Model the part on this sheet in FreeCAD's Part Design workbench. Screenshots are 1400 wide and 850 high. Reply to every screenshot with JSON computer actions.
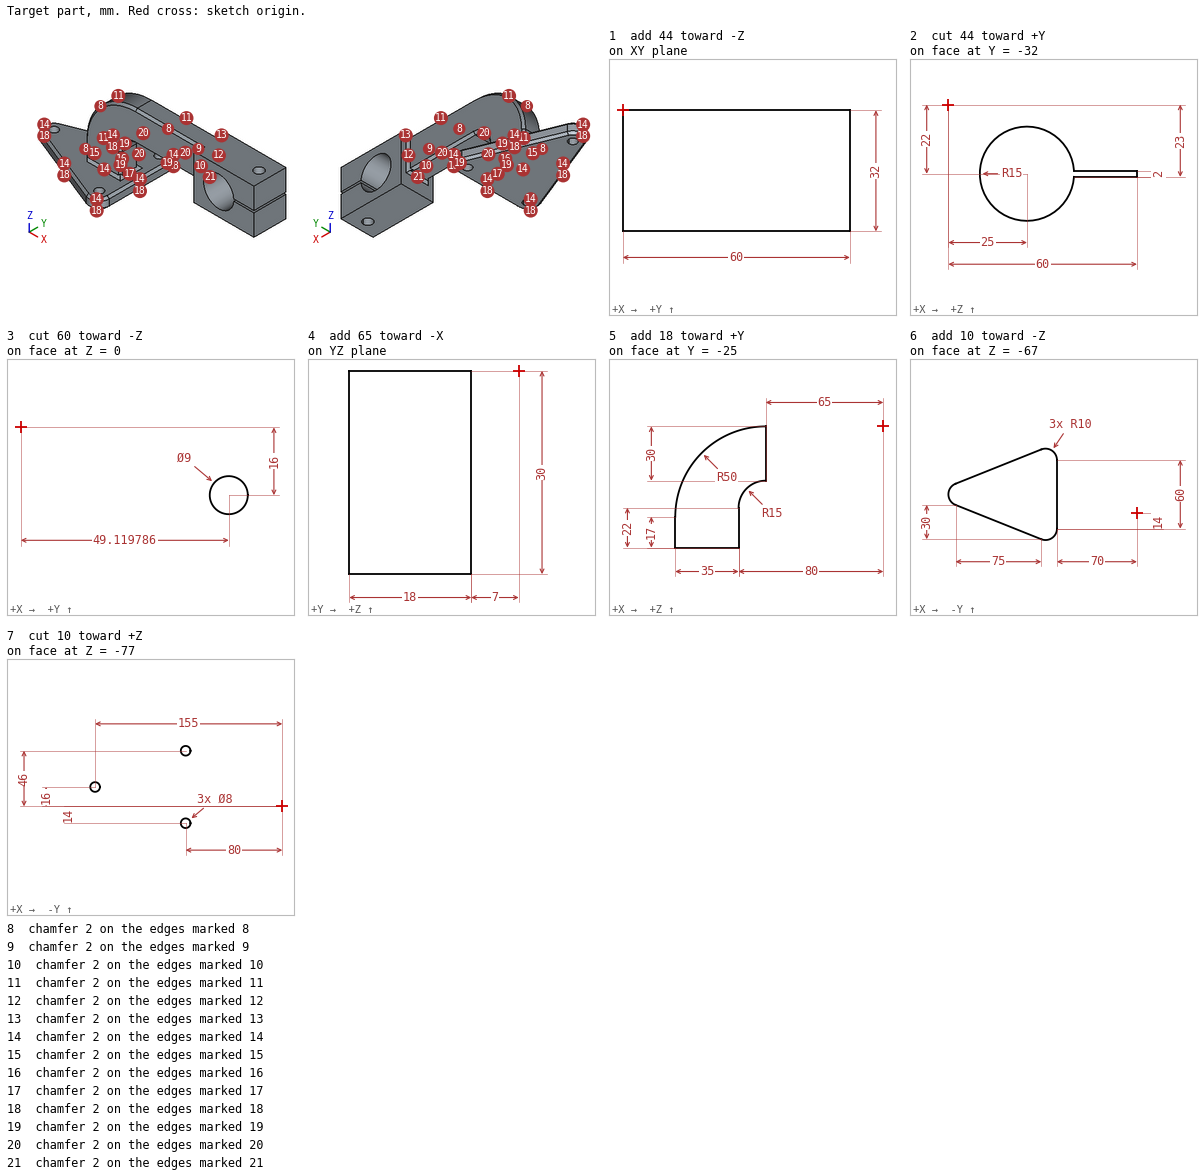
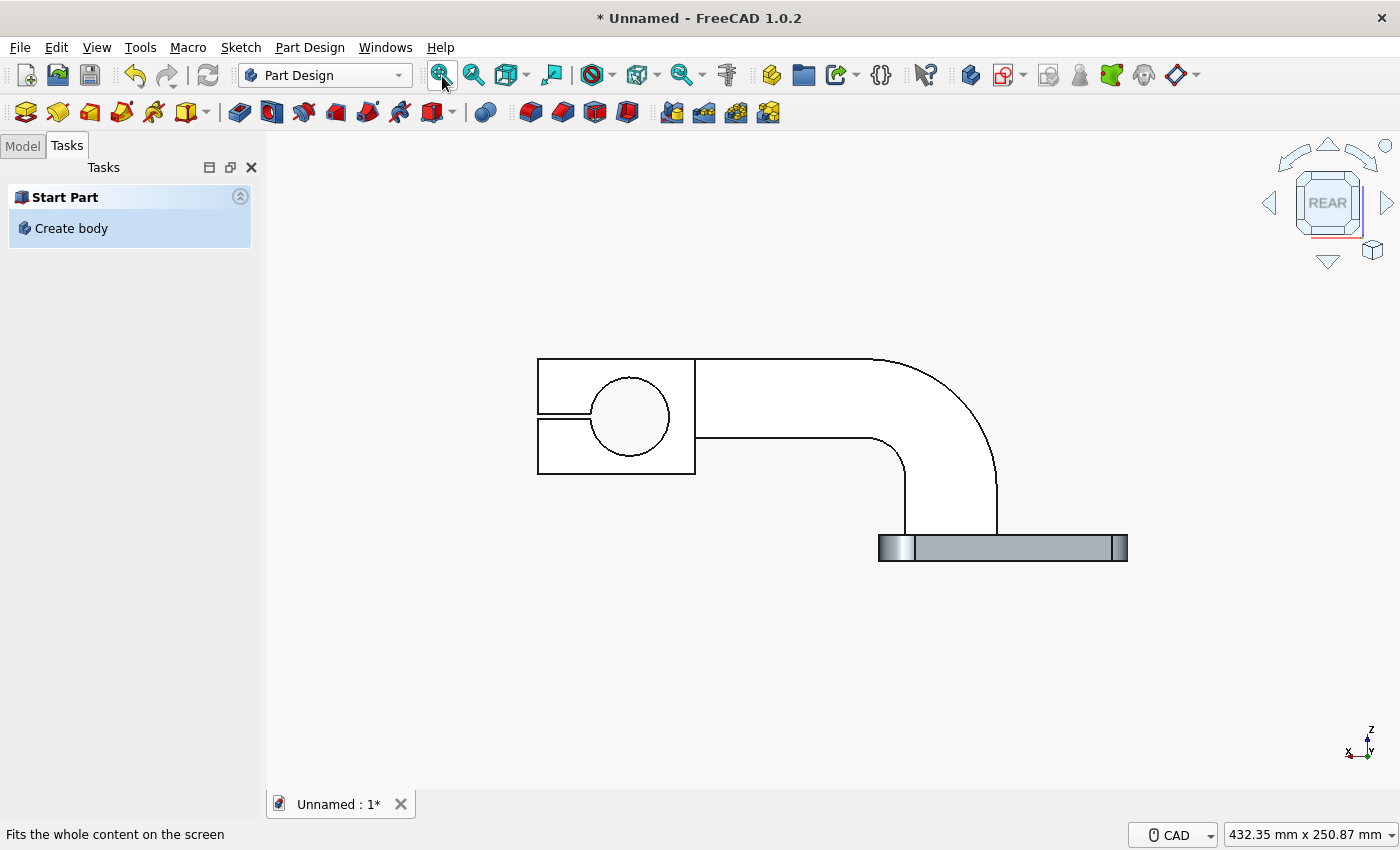
{"action": "key", "text": "6"}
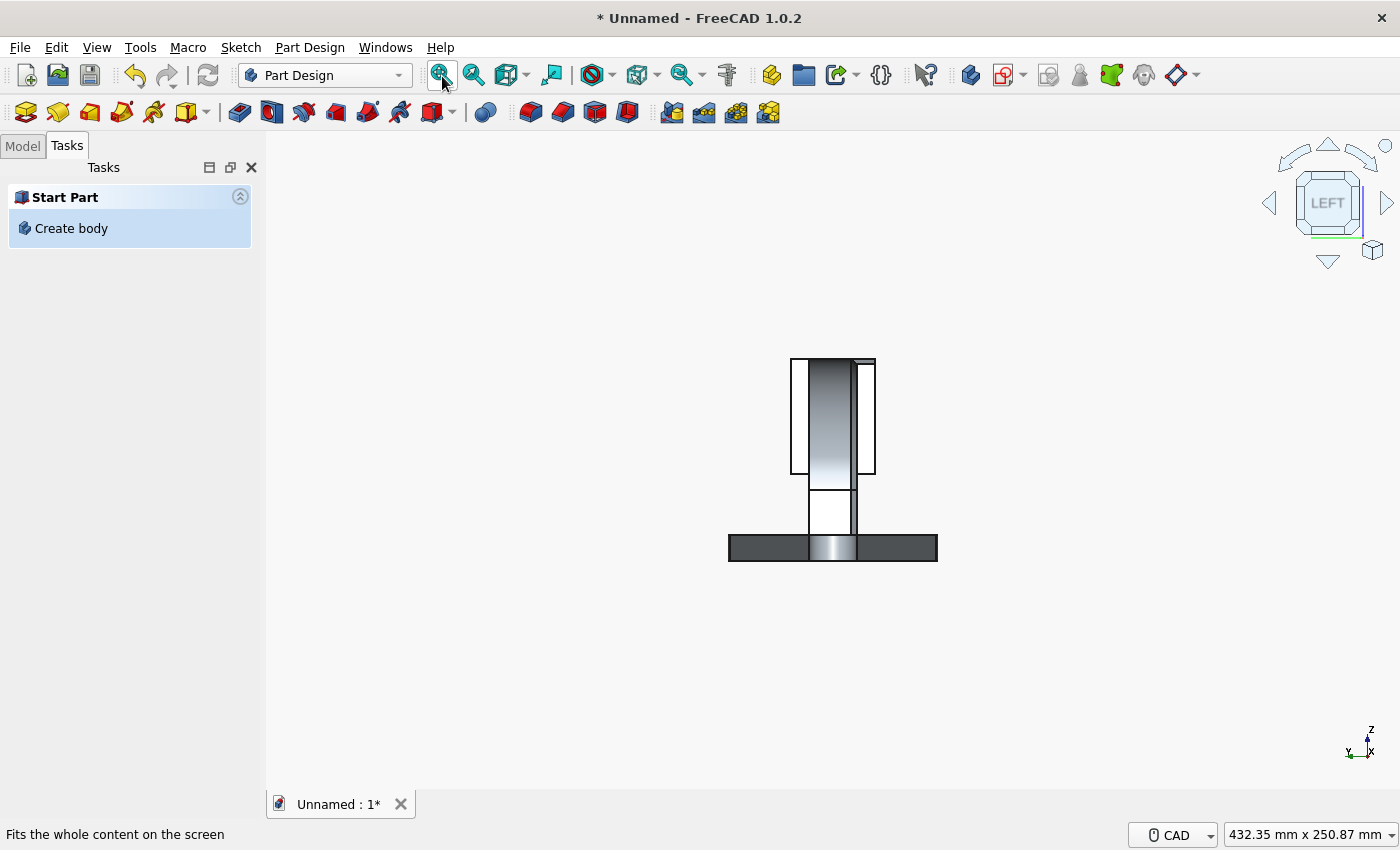
{"action": "left_click", "coordinate": [442, 76]}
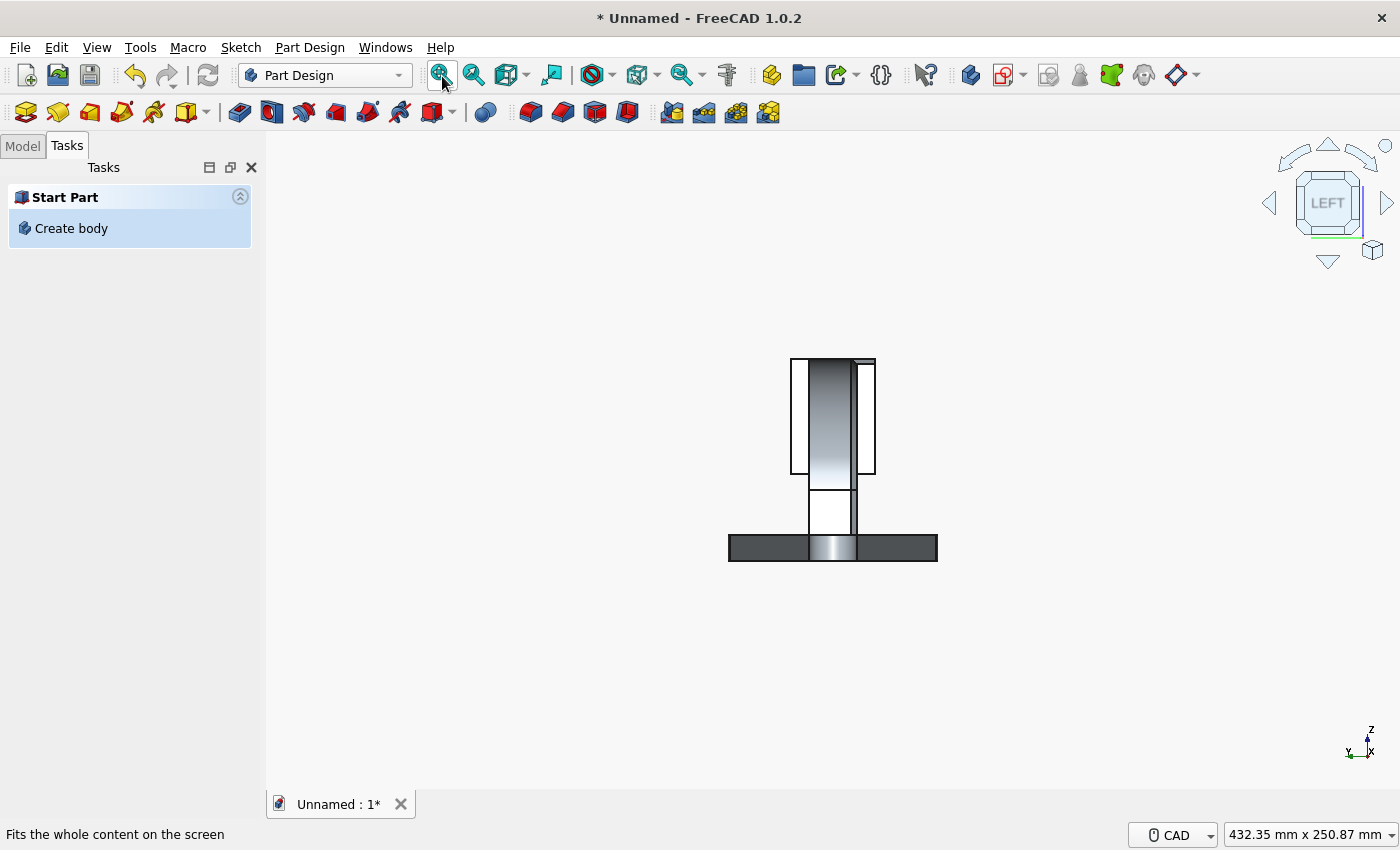
{"action": "key", "text": "v 3"}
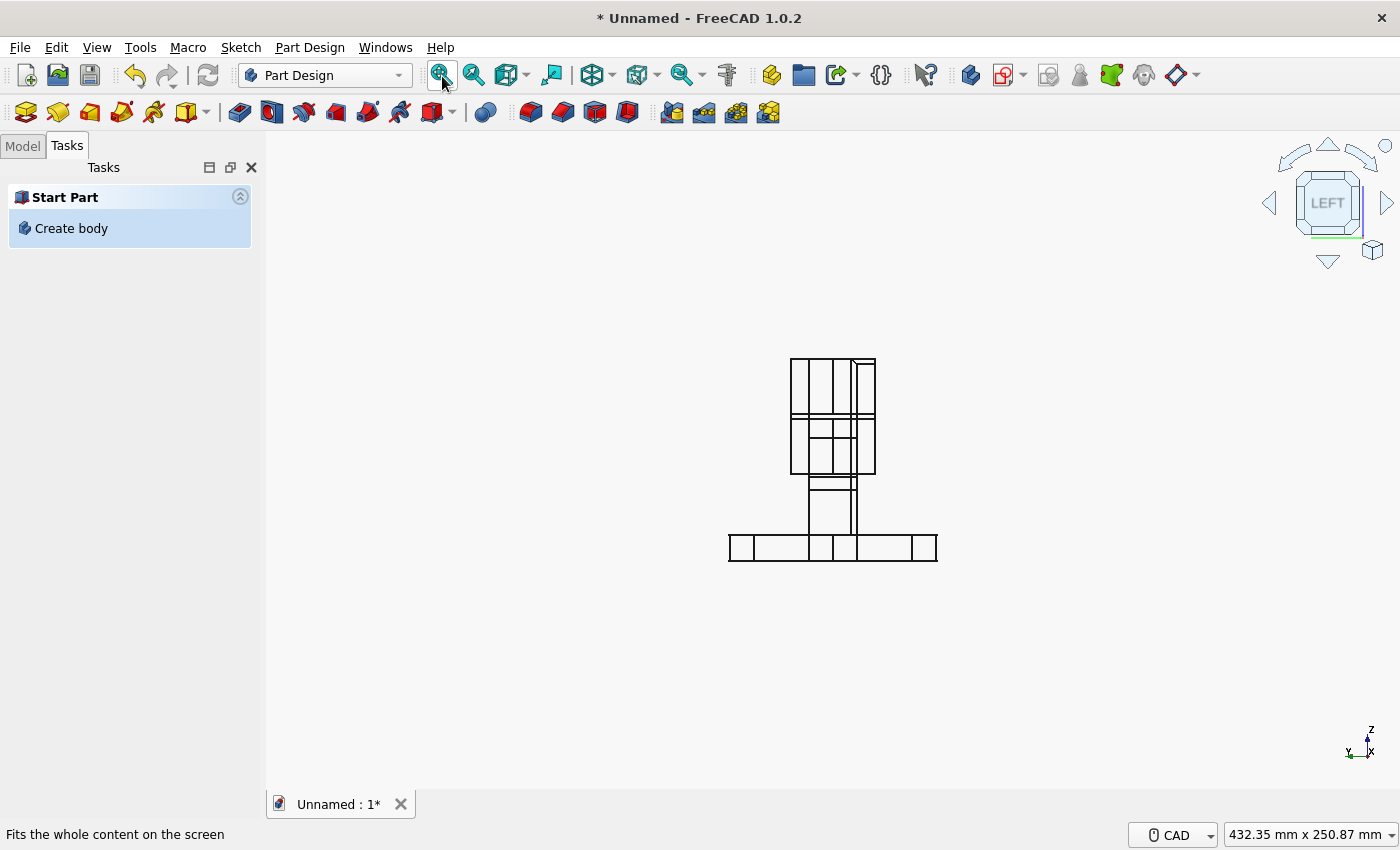
{"action": "key", "text": "0"}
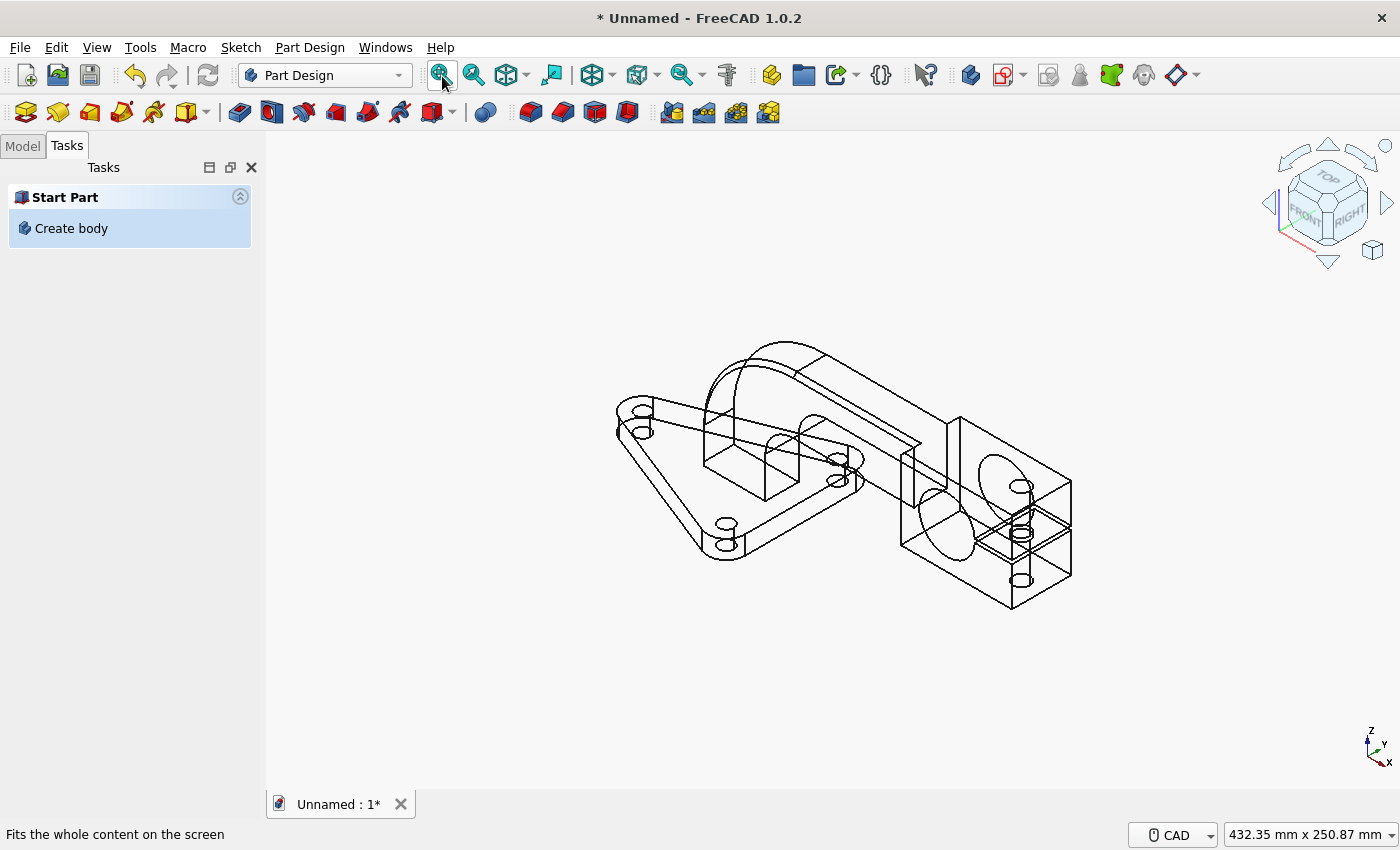
{"action": "left_click", "coordinate": [914, 477]}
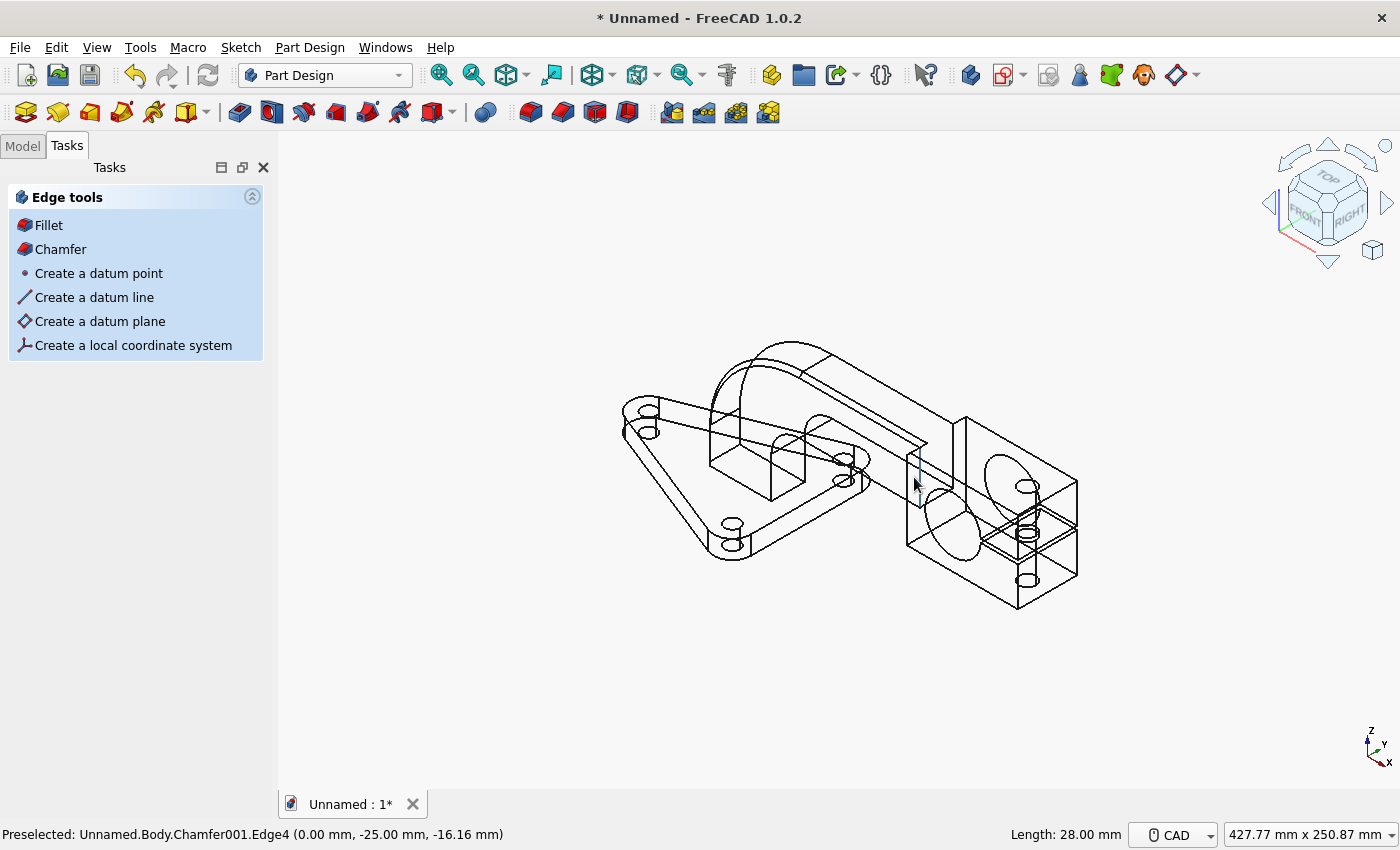
{"action": "key", "text": "v 1"}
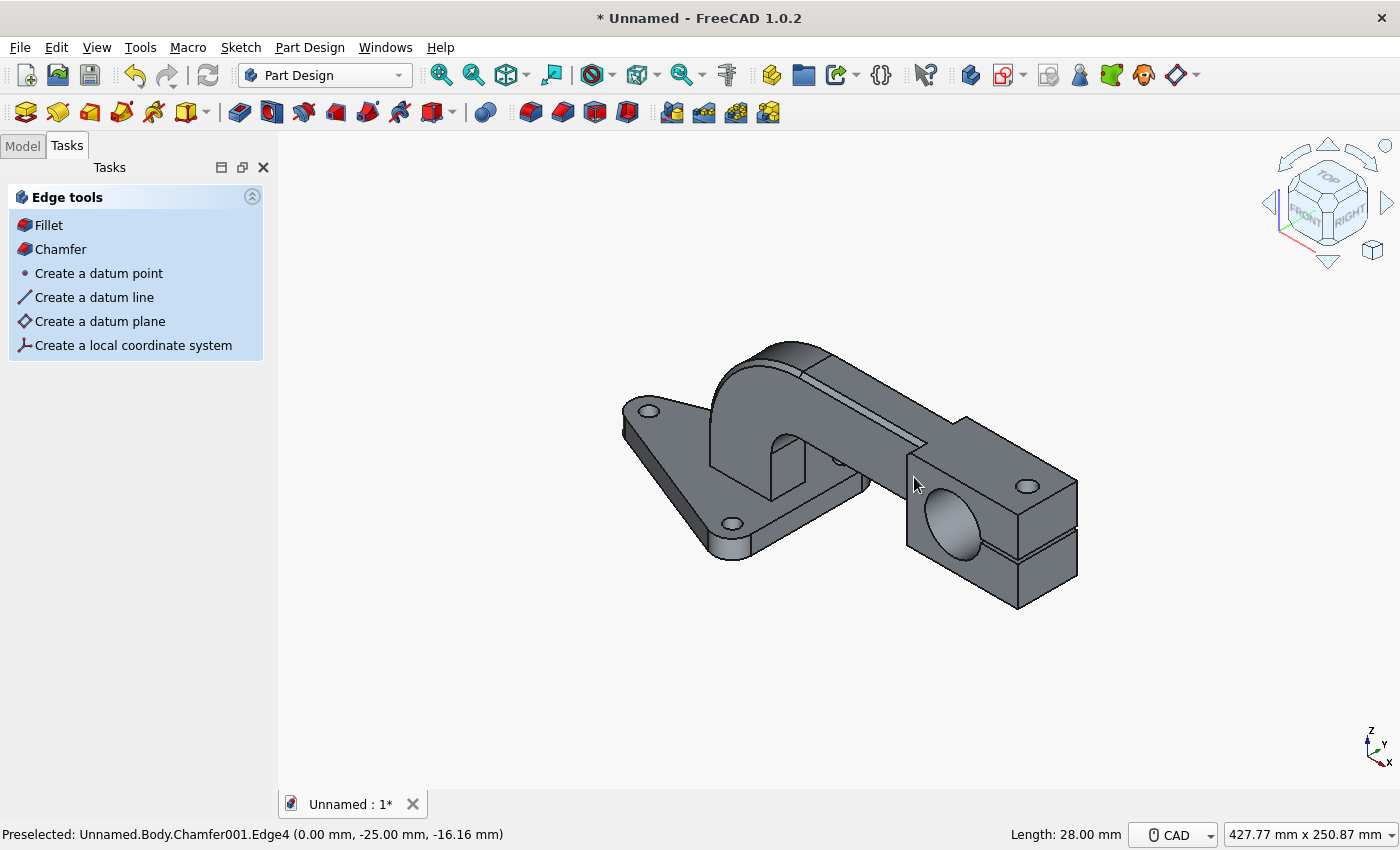
{"action": "left_click", "coordinate": [564, 112]}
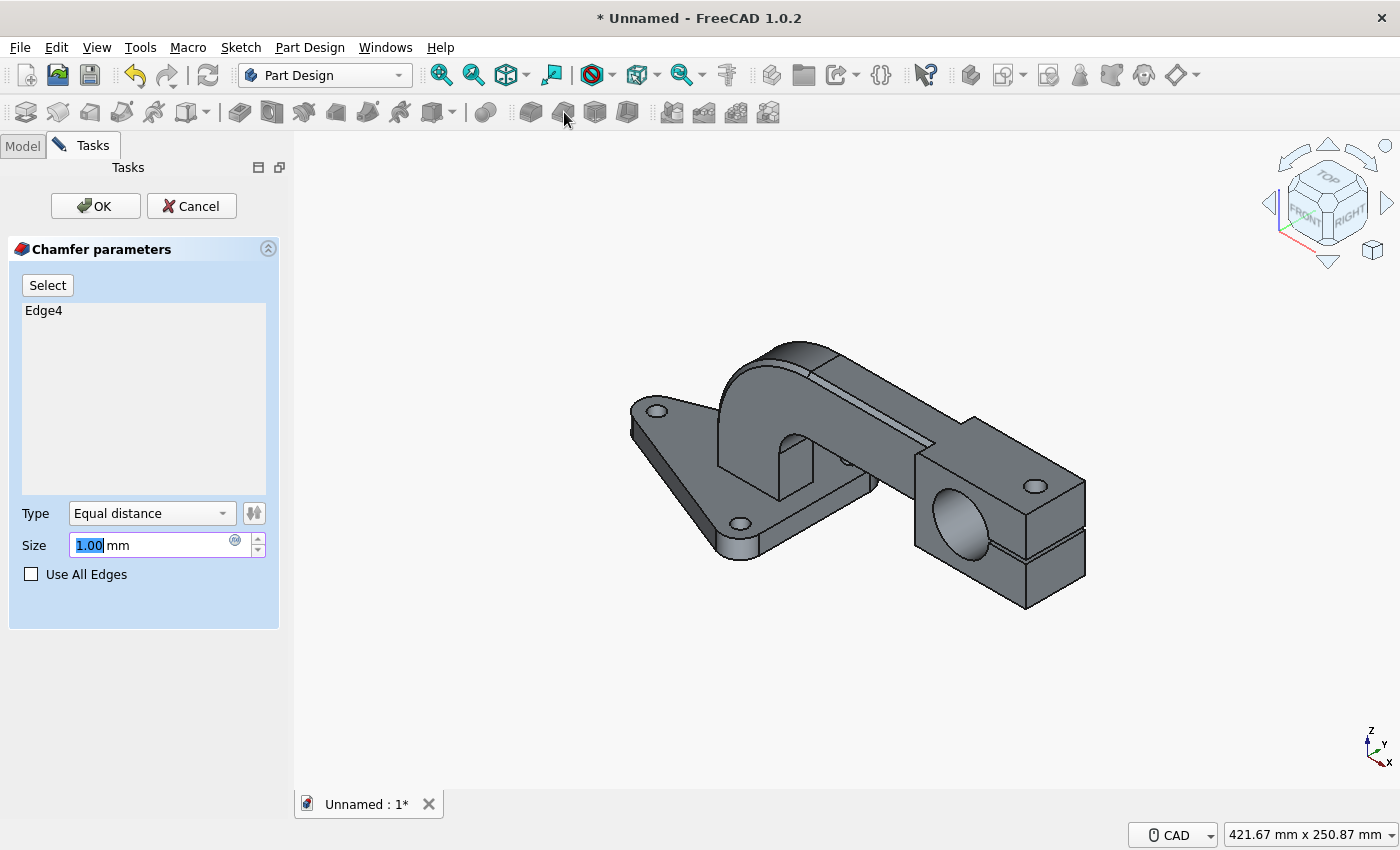
{"action": "type", "text": "2"}
{"action": "key", "text": "Tab"}